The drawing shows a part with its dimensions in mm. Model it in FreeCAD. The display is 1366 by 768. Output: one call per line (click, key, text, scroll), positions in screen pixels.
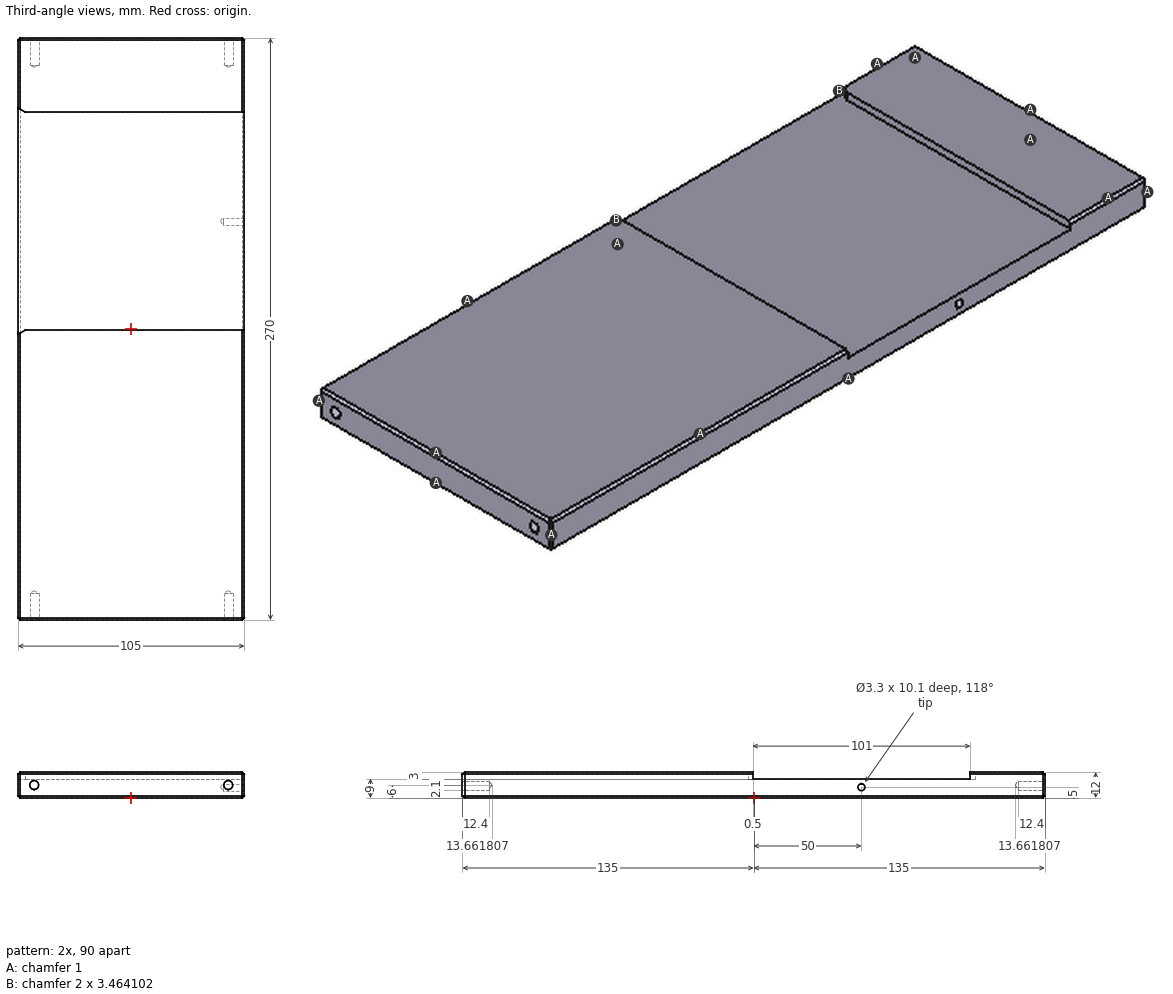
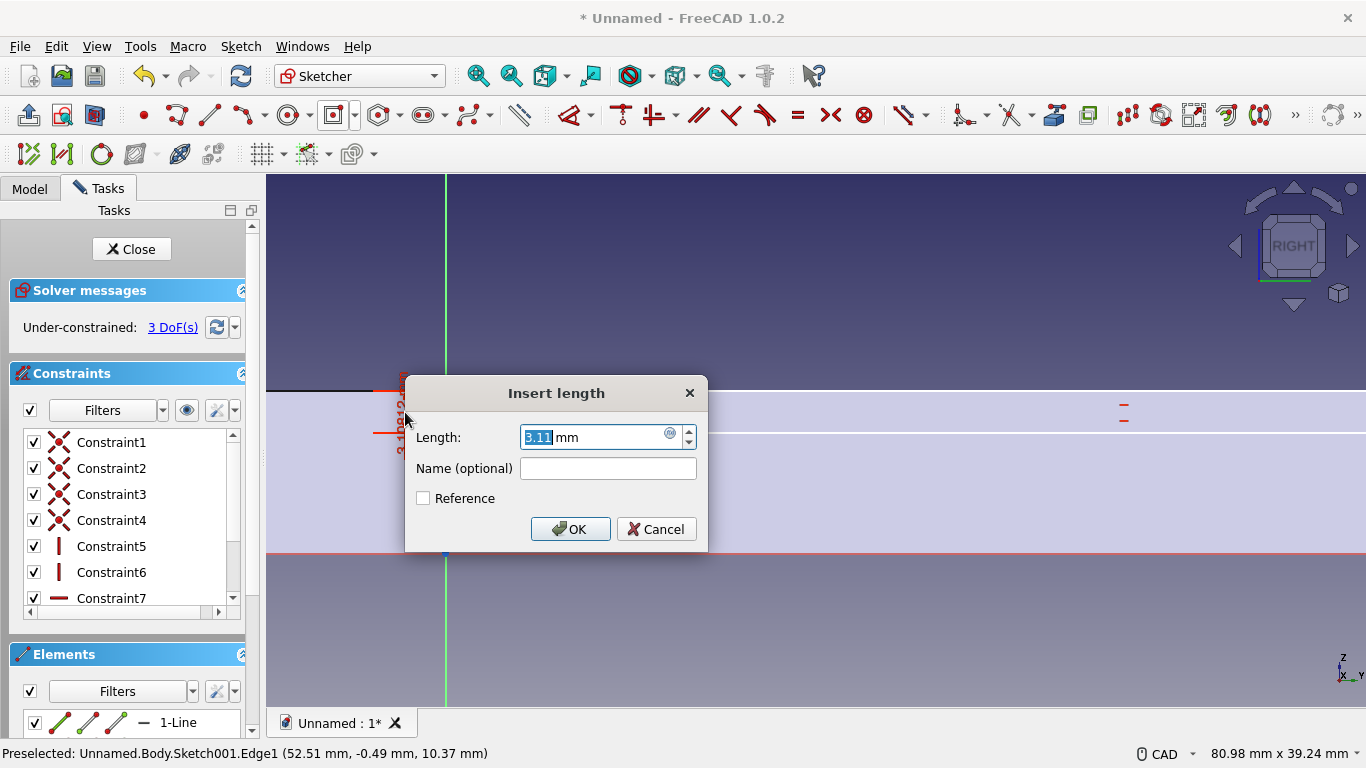
text(3)
key(Return)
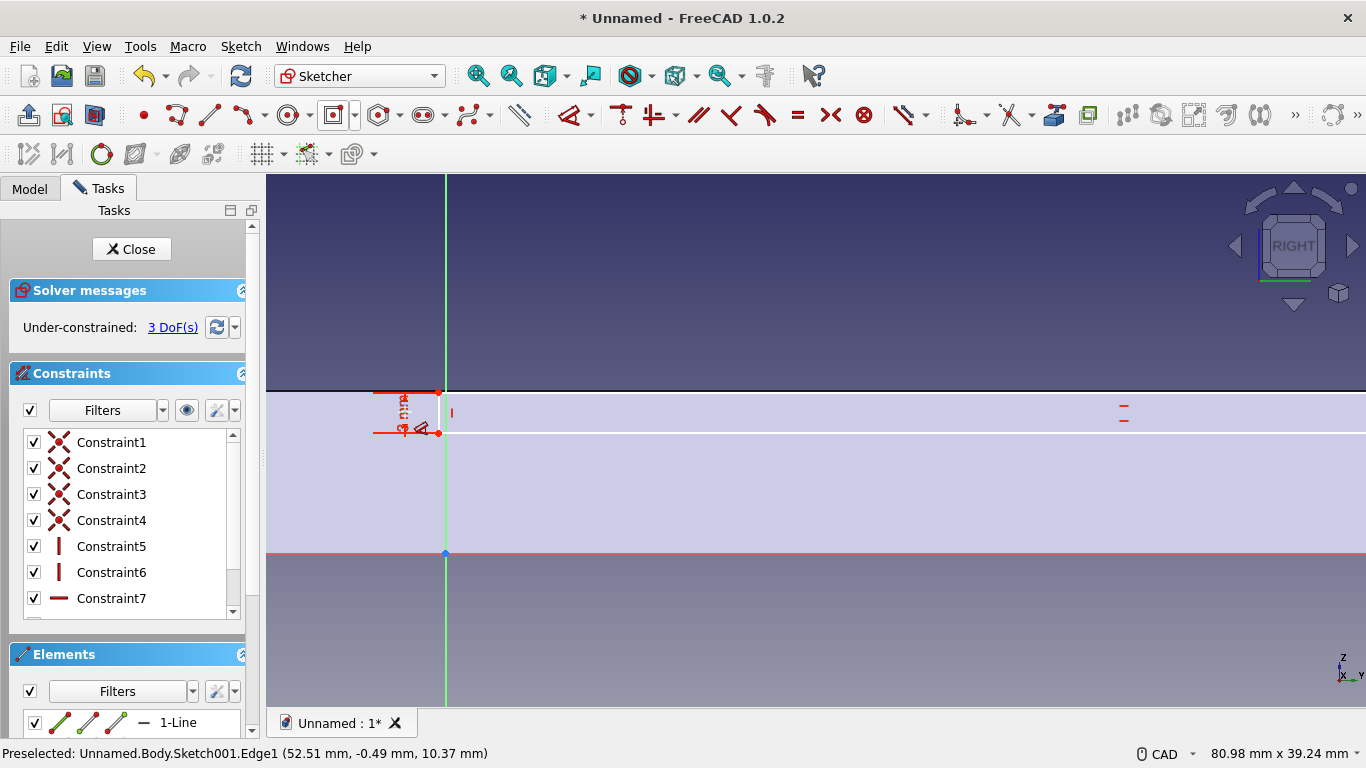
click(439, 433)
click(405, 494)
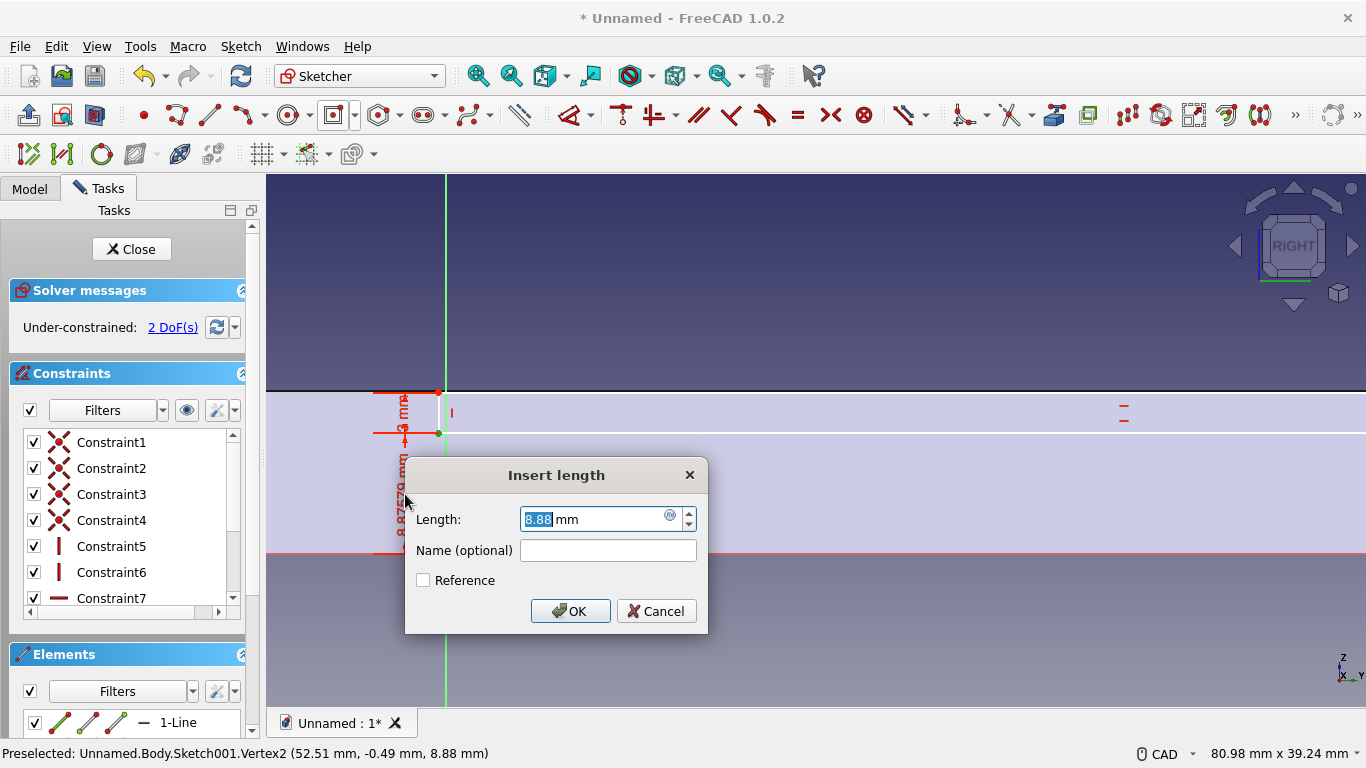
text(9)
key(Return)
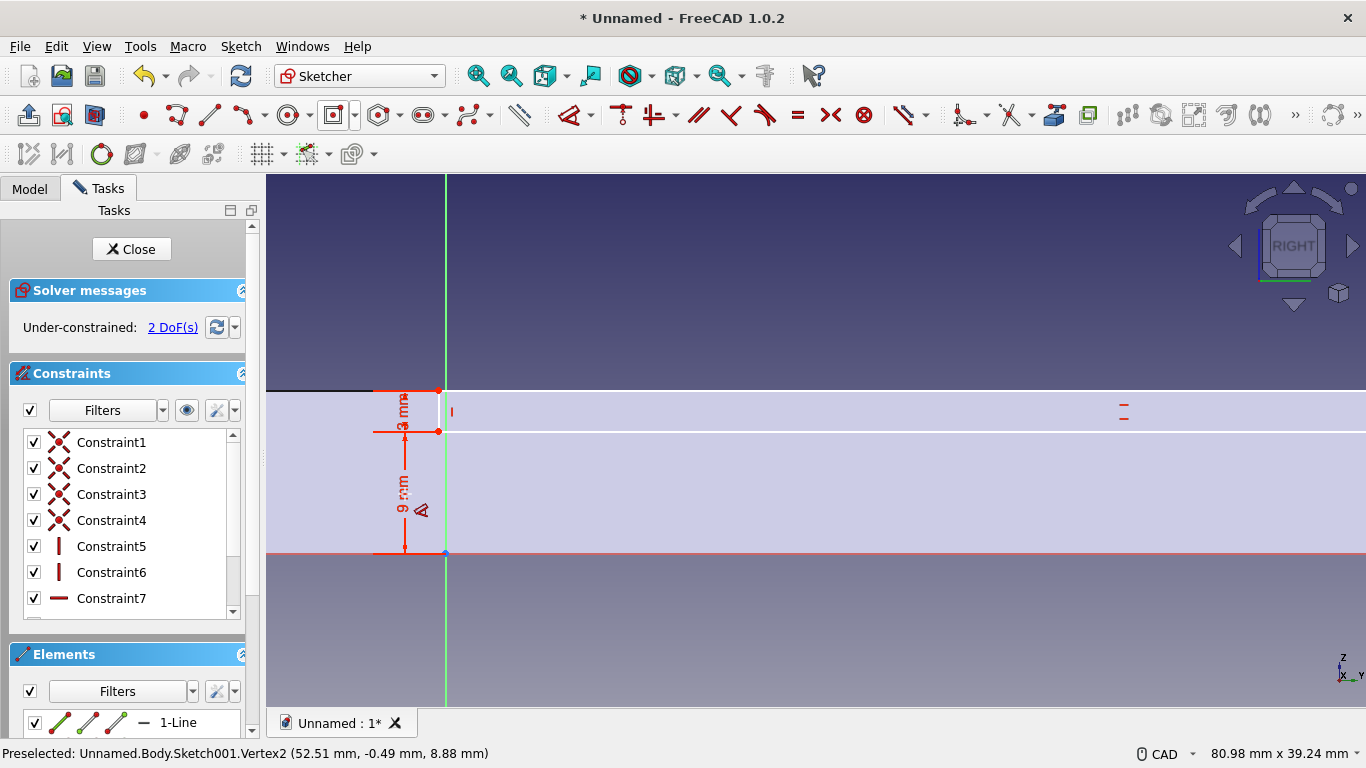
click(851, 432)
click(820, 466)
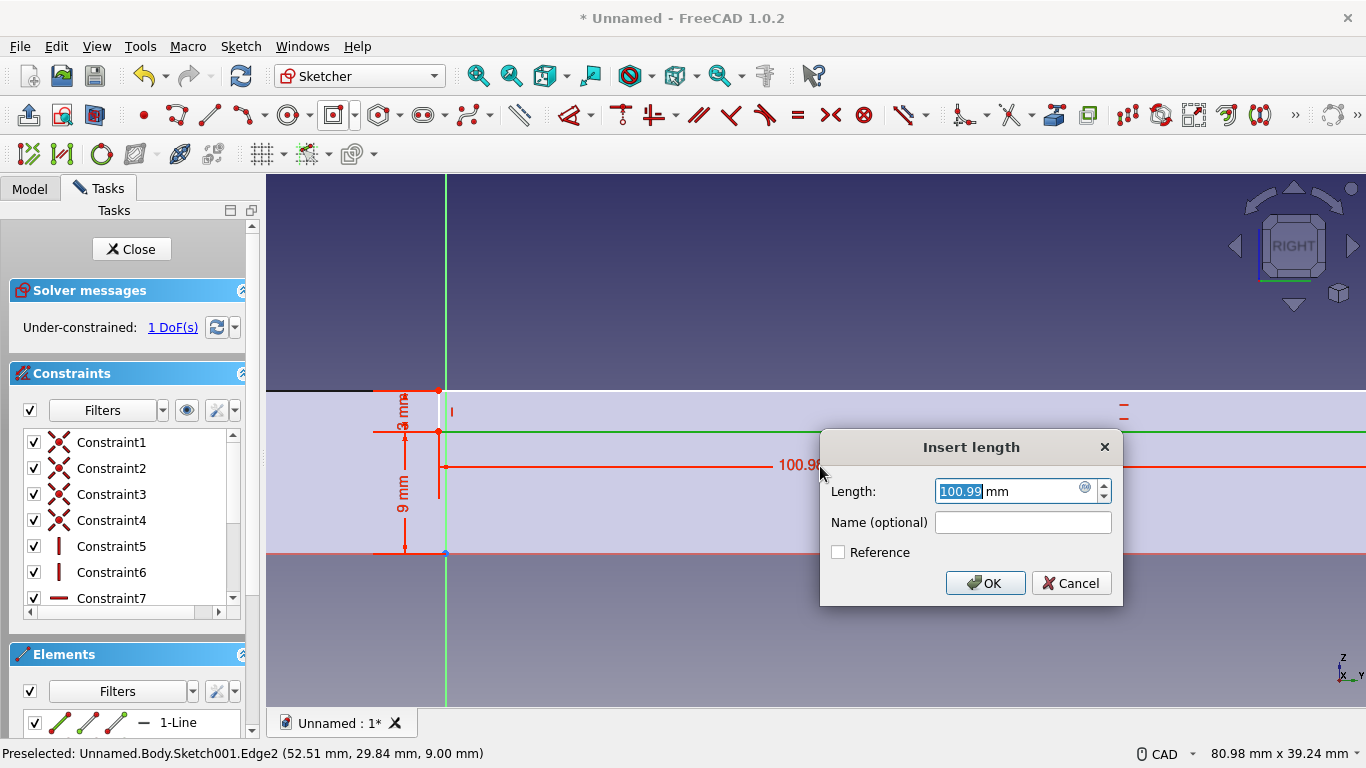
text(101)
key(Return)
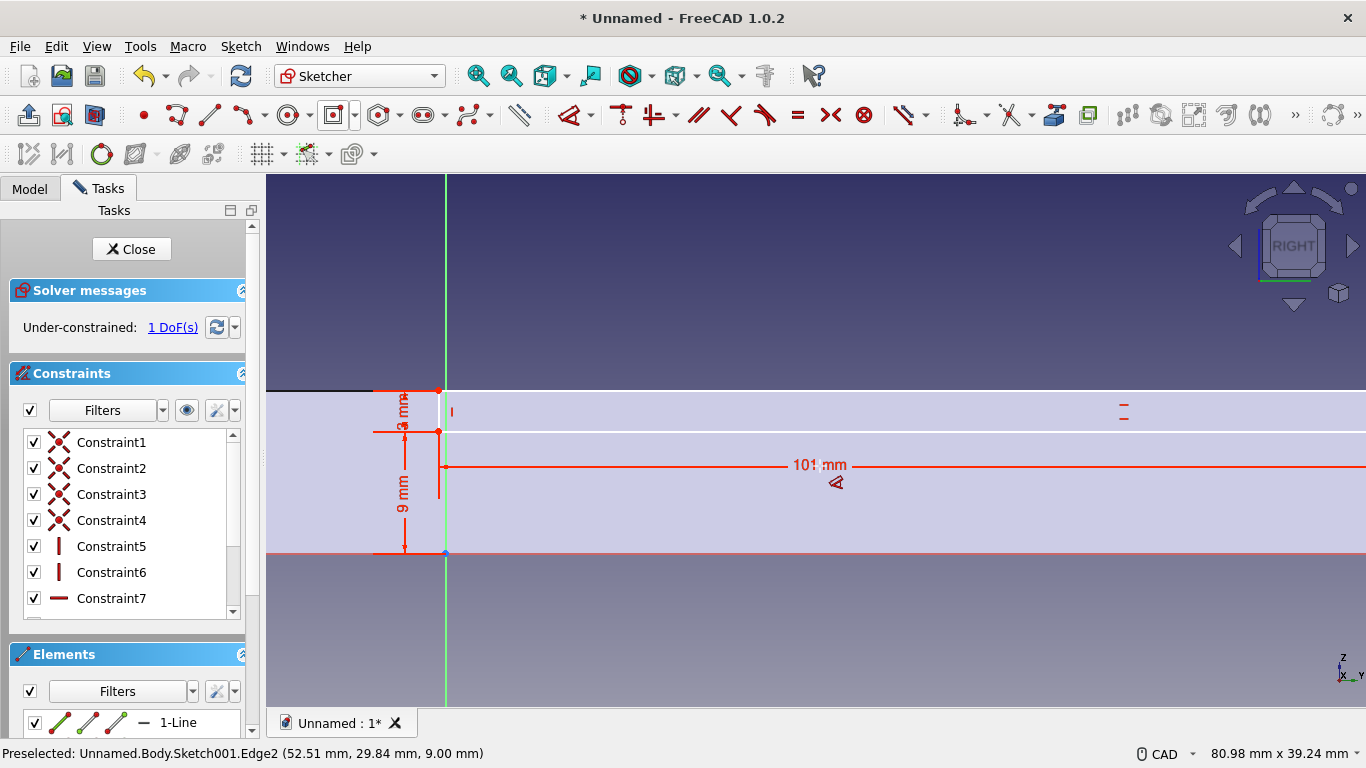
scroll(439, 391, up, 9)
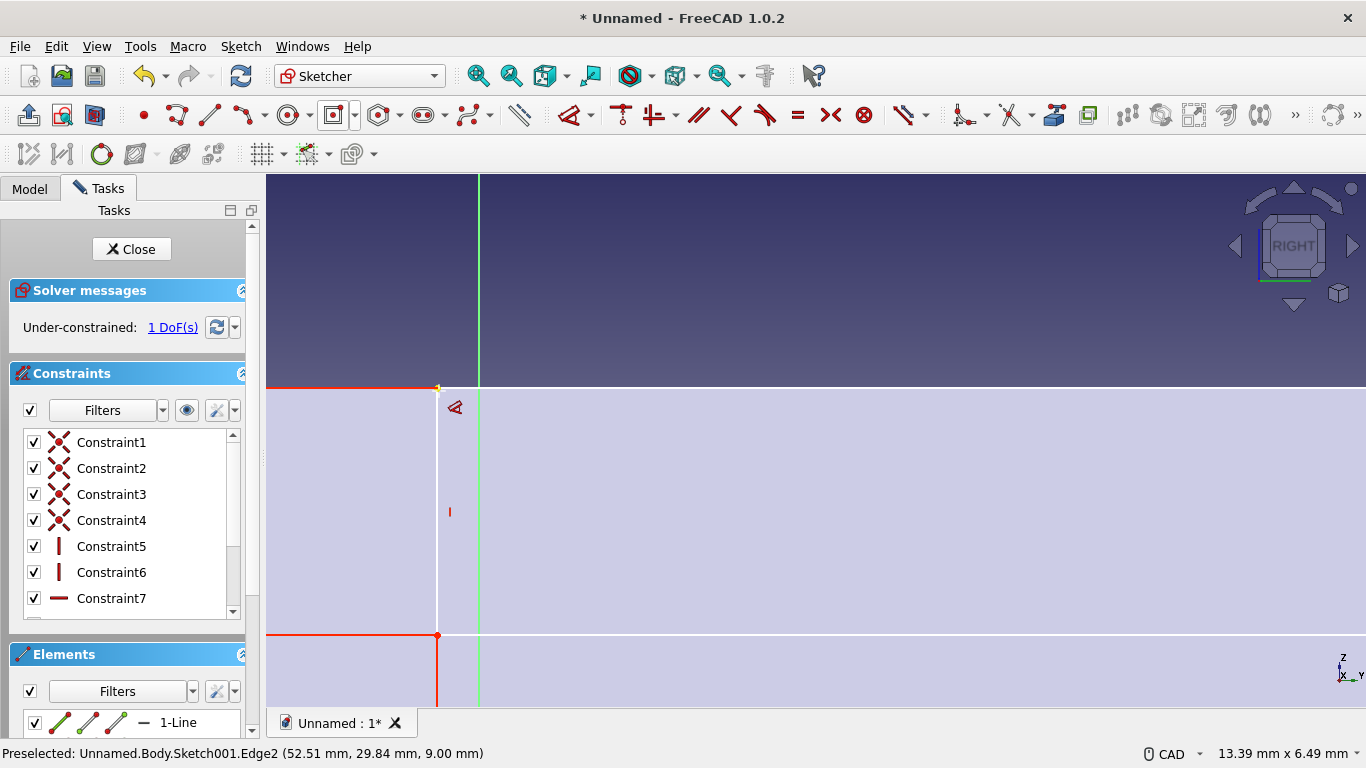
click(437, 388)
click(458, 354)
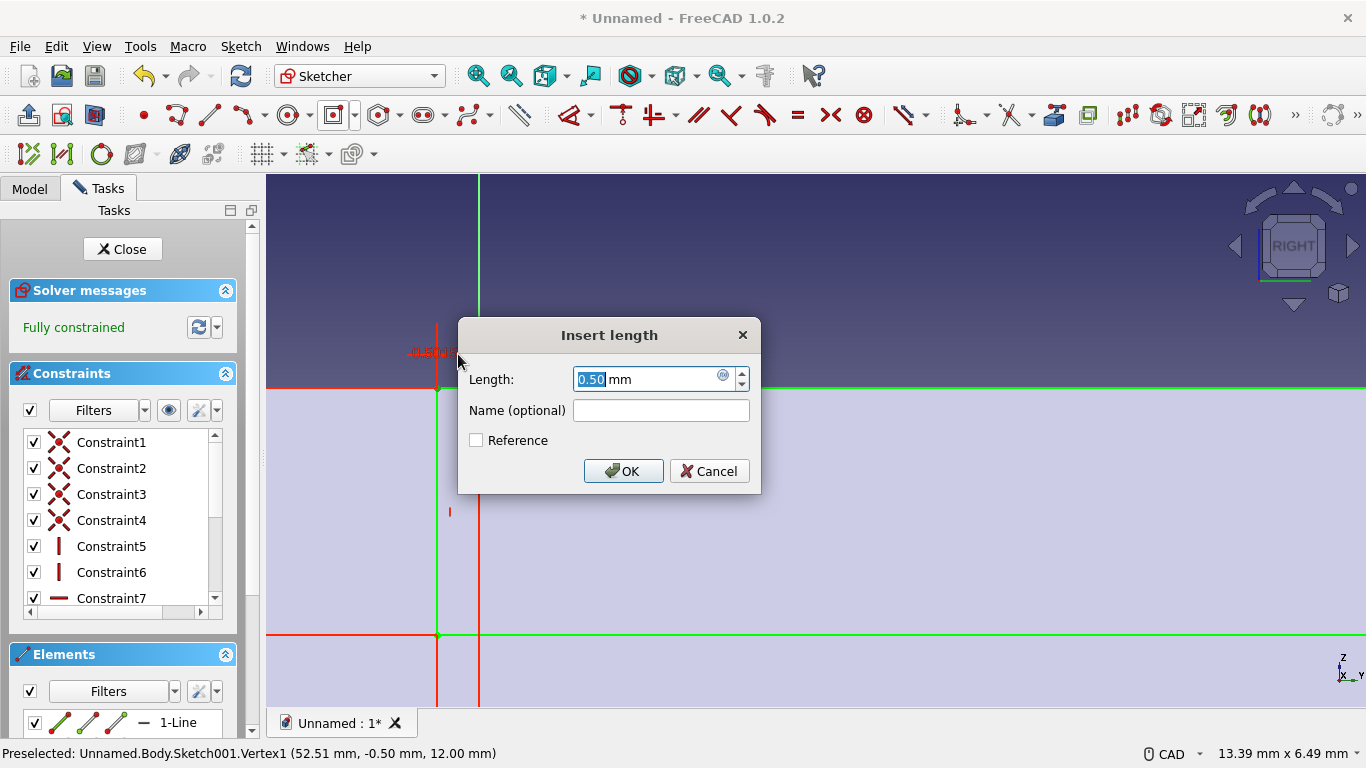
text(0.5)
key(Return)
key(Escape)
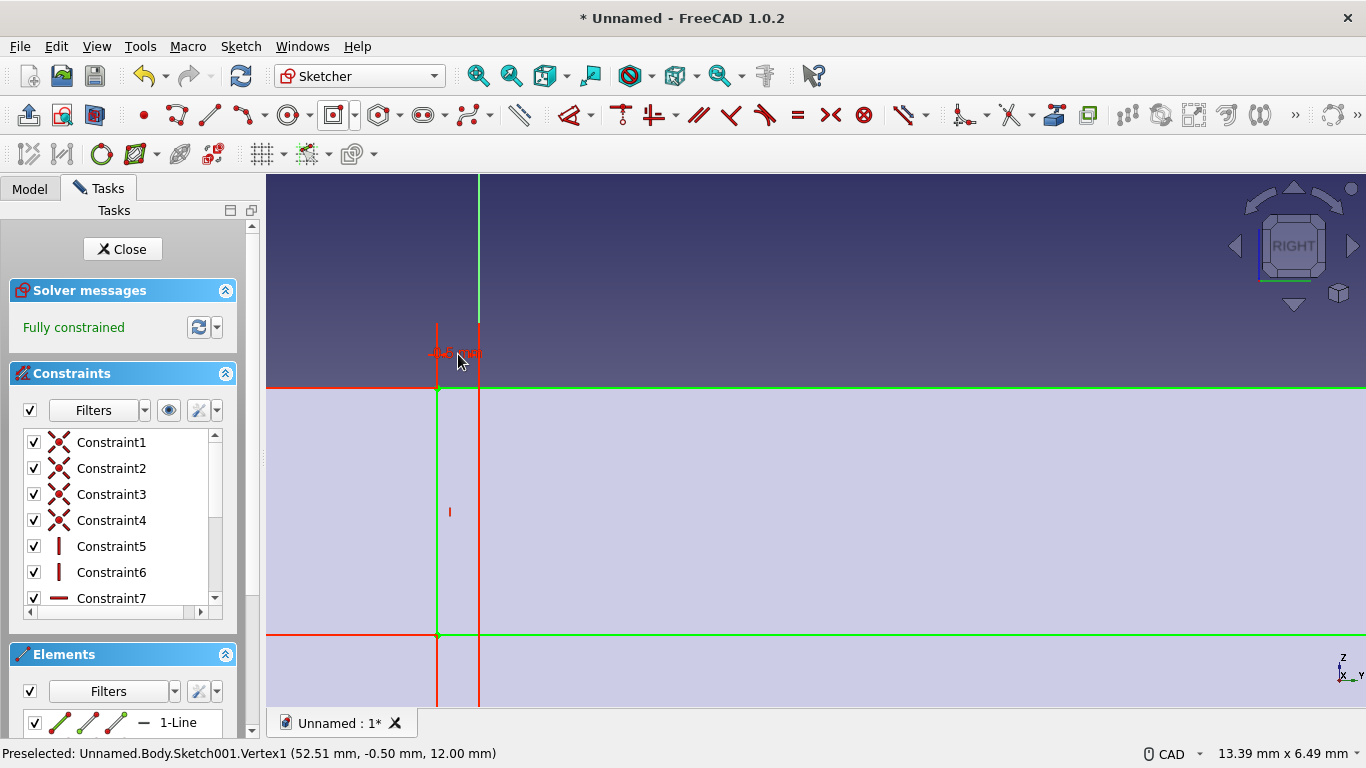
click(123, 249)